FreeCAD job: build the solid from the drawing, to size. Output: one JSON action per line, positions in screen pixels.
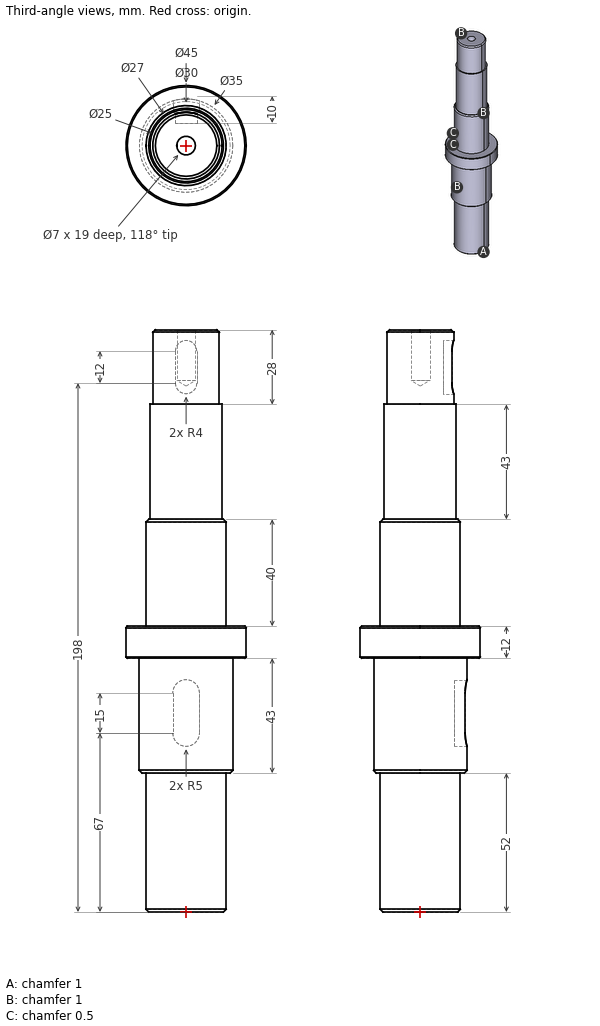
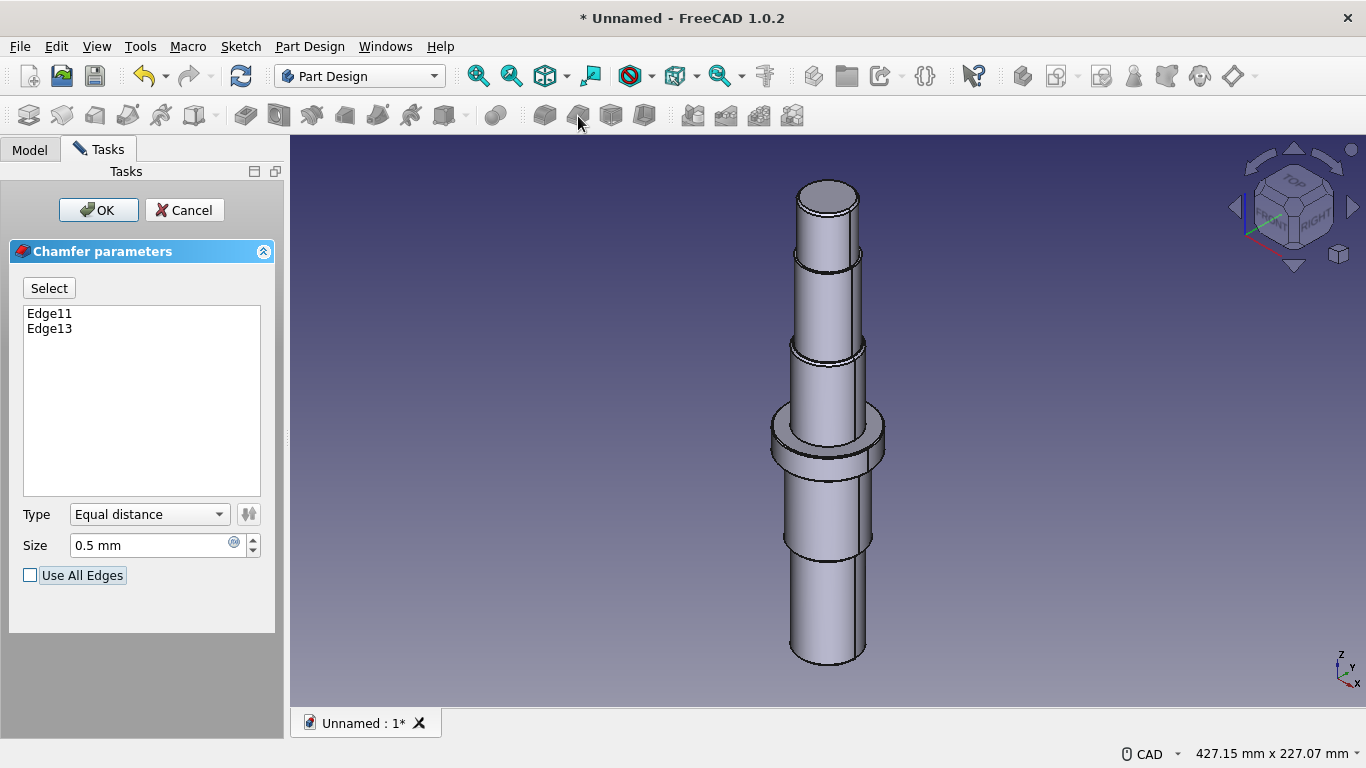
{"action": "left_click", "coordinate": [99, 210]}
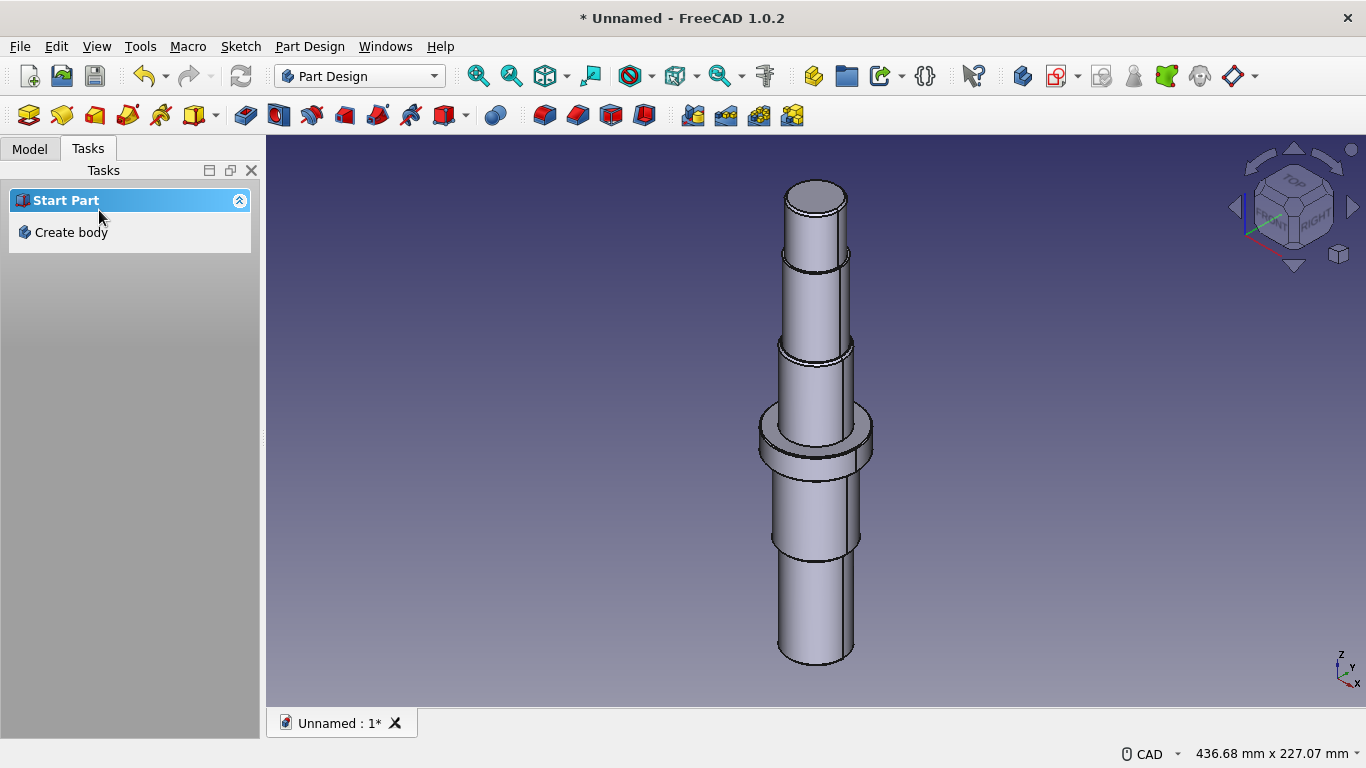
{"action": "left_click", "coordinate": [30, 148]}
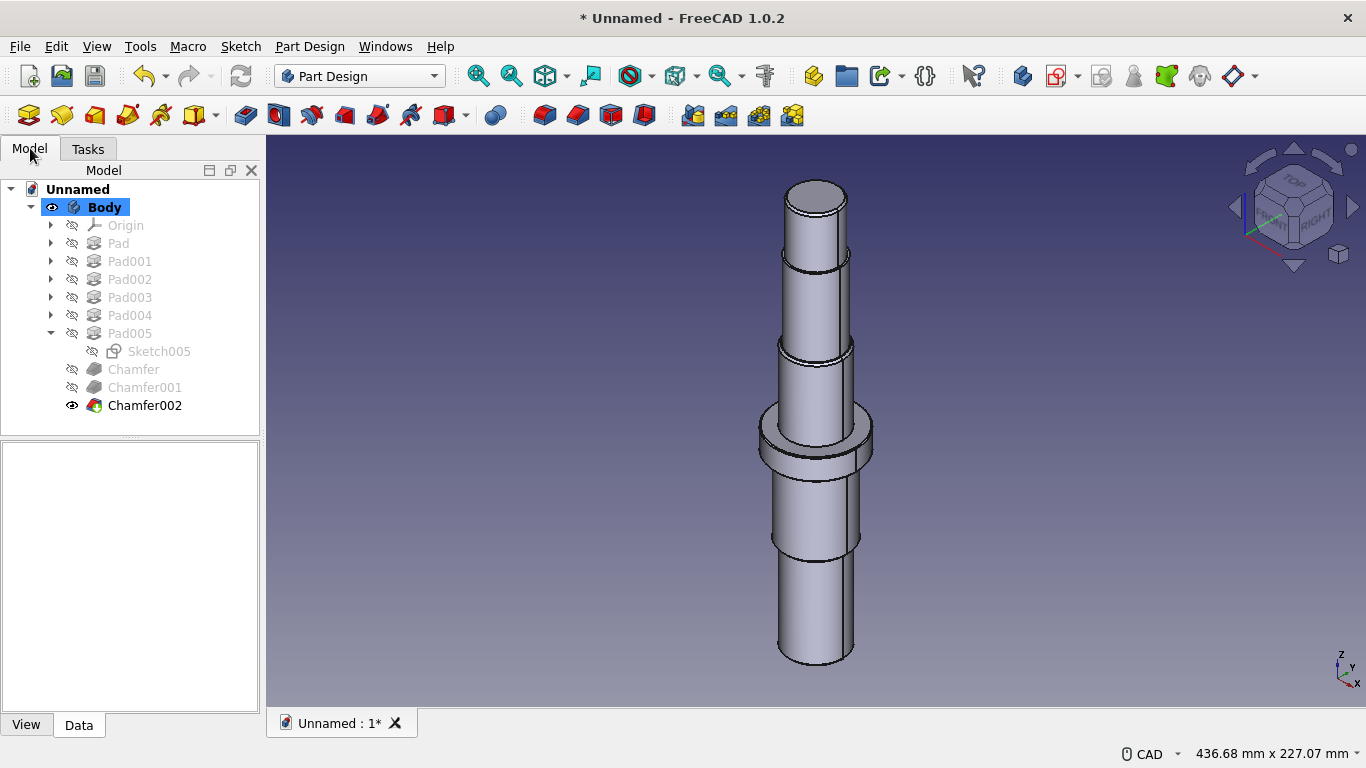
{"action": "left_click", "coordinate": [51, 225]}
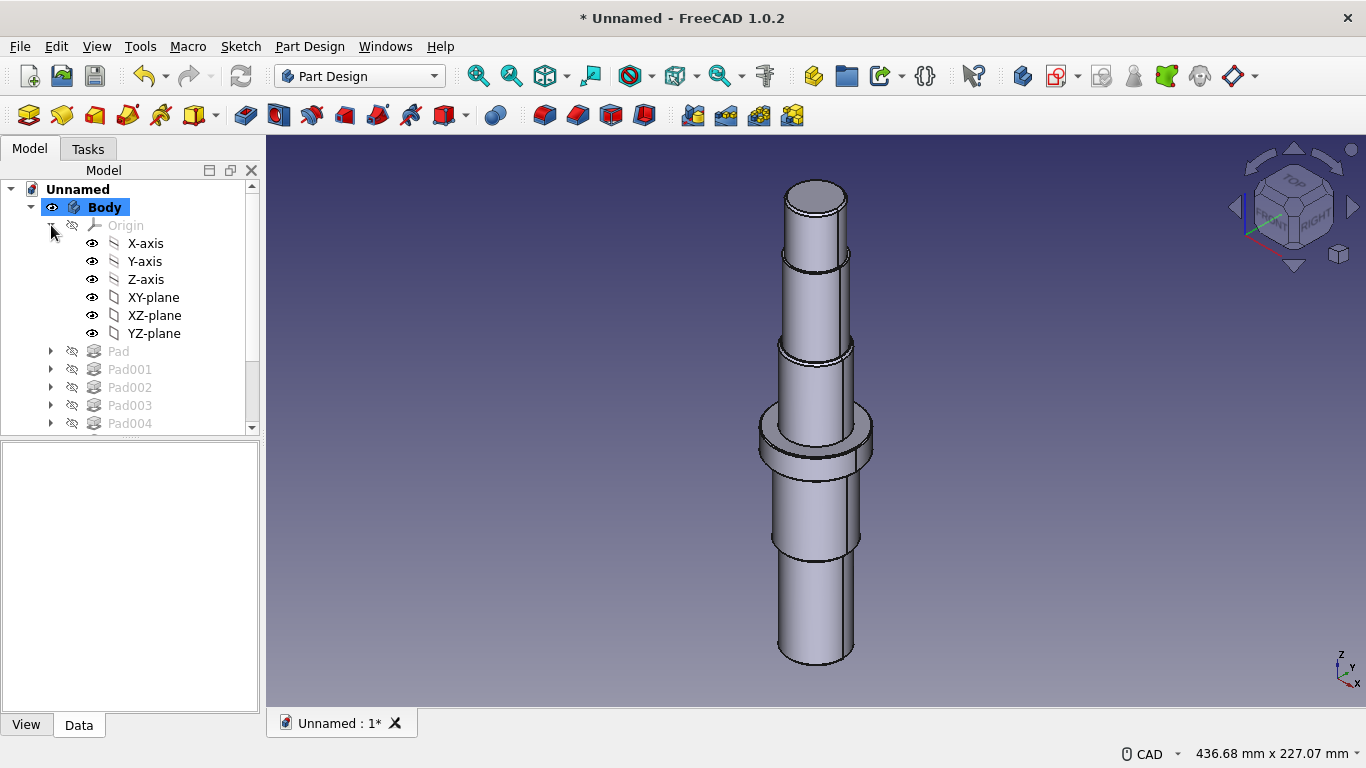
{"action": "left_click", "coordinate": [137, 315]}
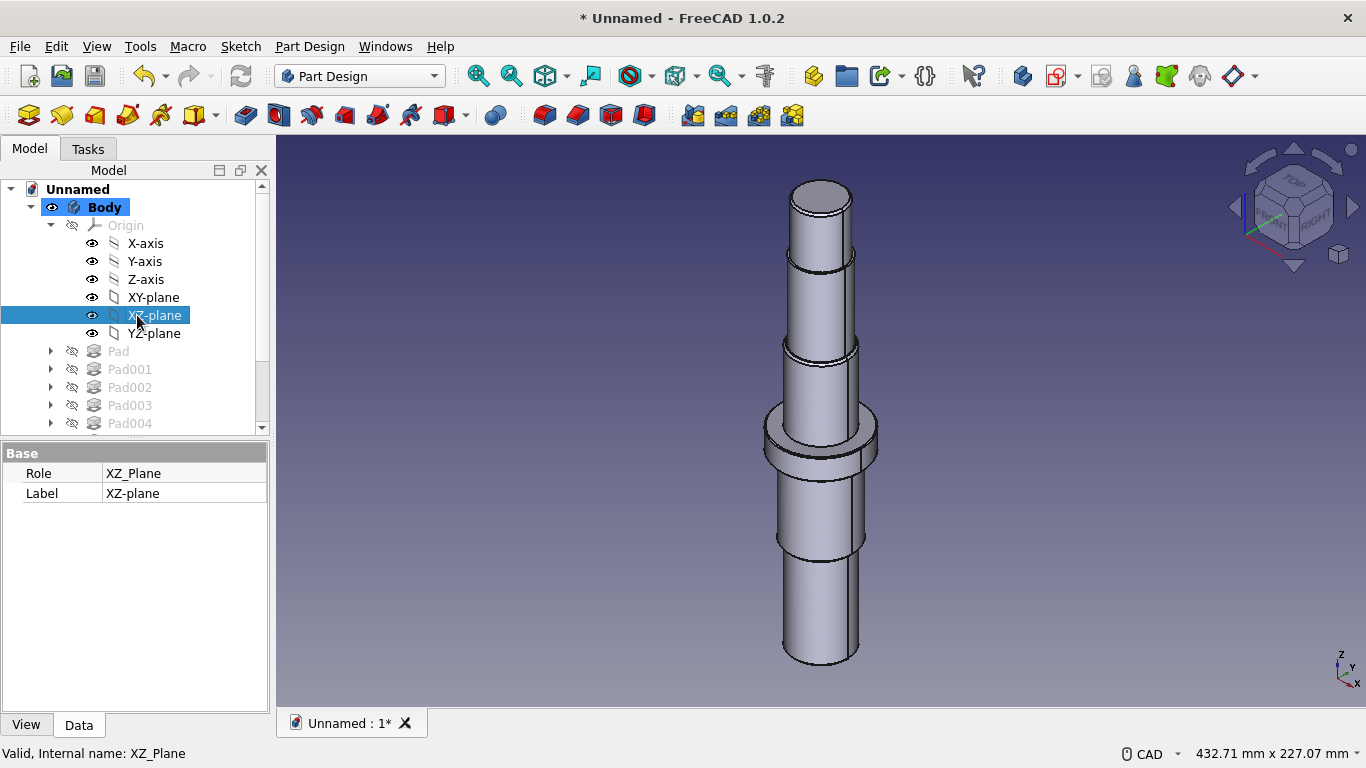
{"action": "left_click", "coordinate": [1232, 76]}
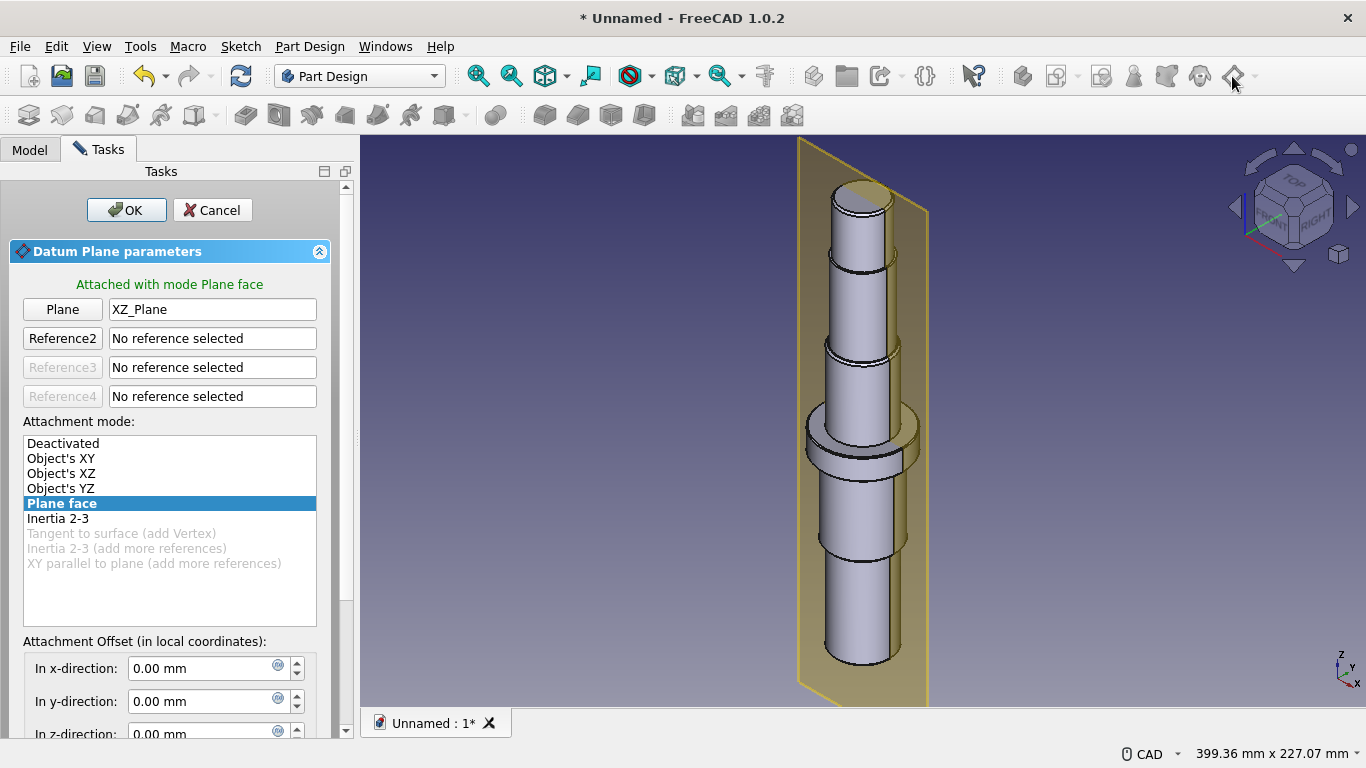
{"action": "scroll", "coordinate": [346, 460], "scroll_direction": "down", "scroll_amount": 2}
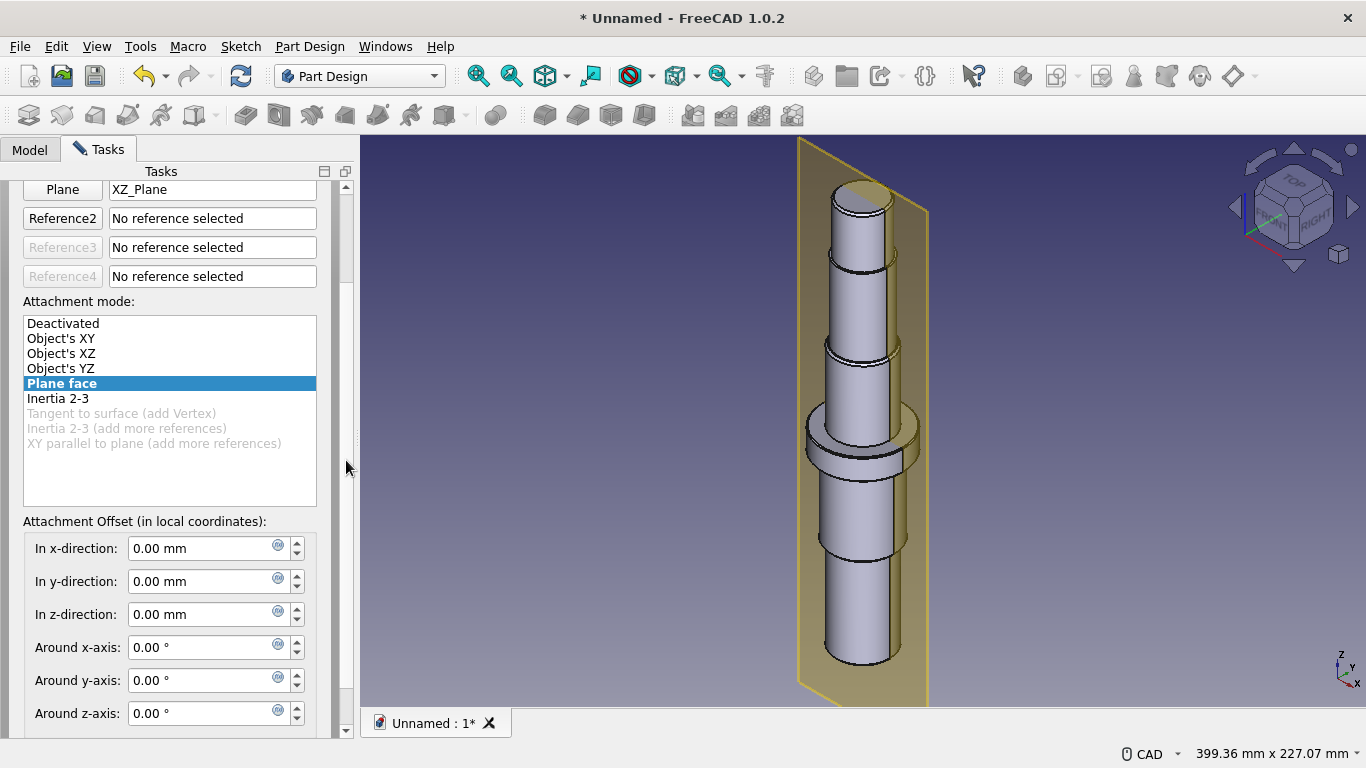
{"action": "triple_click", "coordinate": [210, 614]}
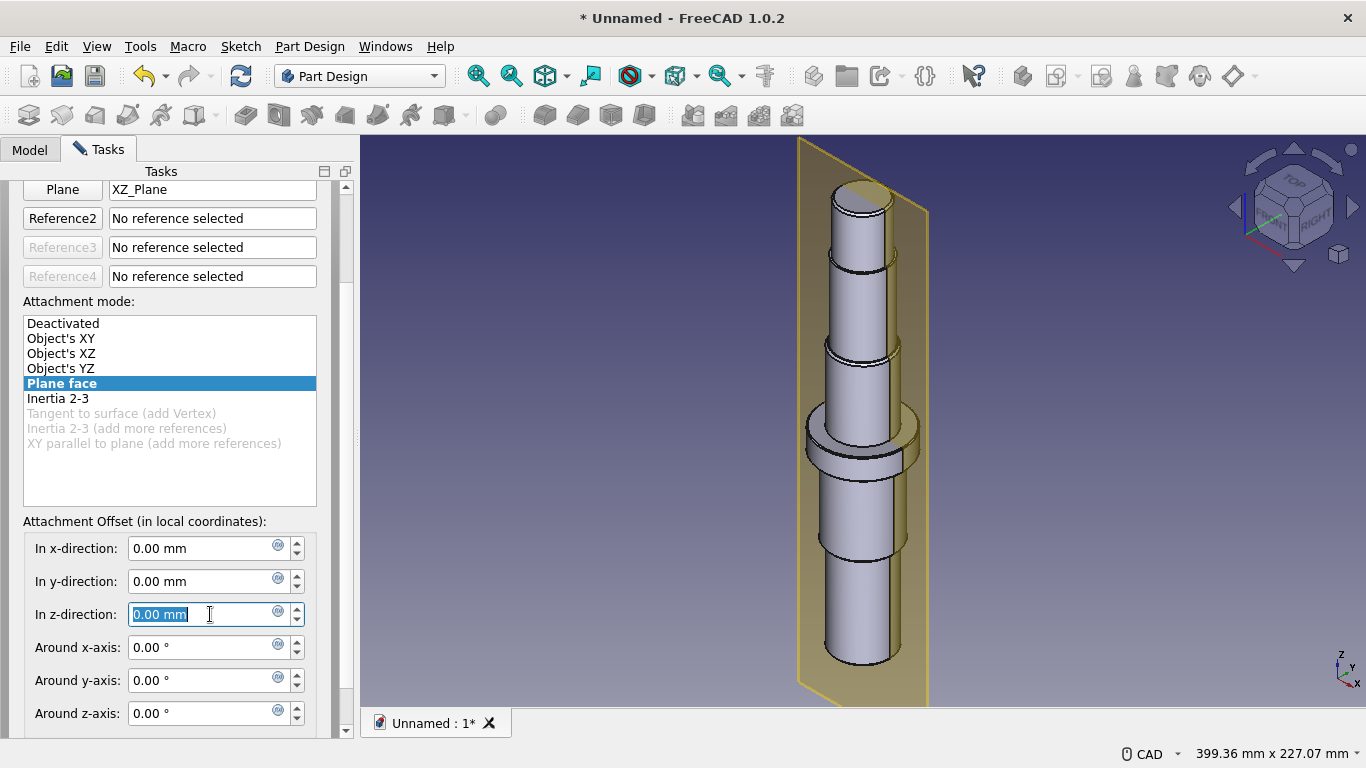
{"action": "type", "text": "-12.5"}
{"action": "key", "text": "Tab"}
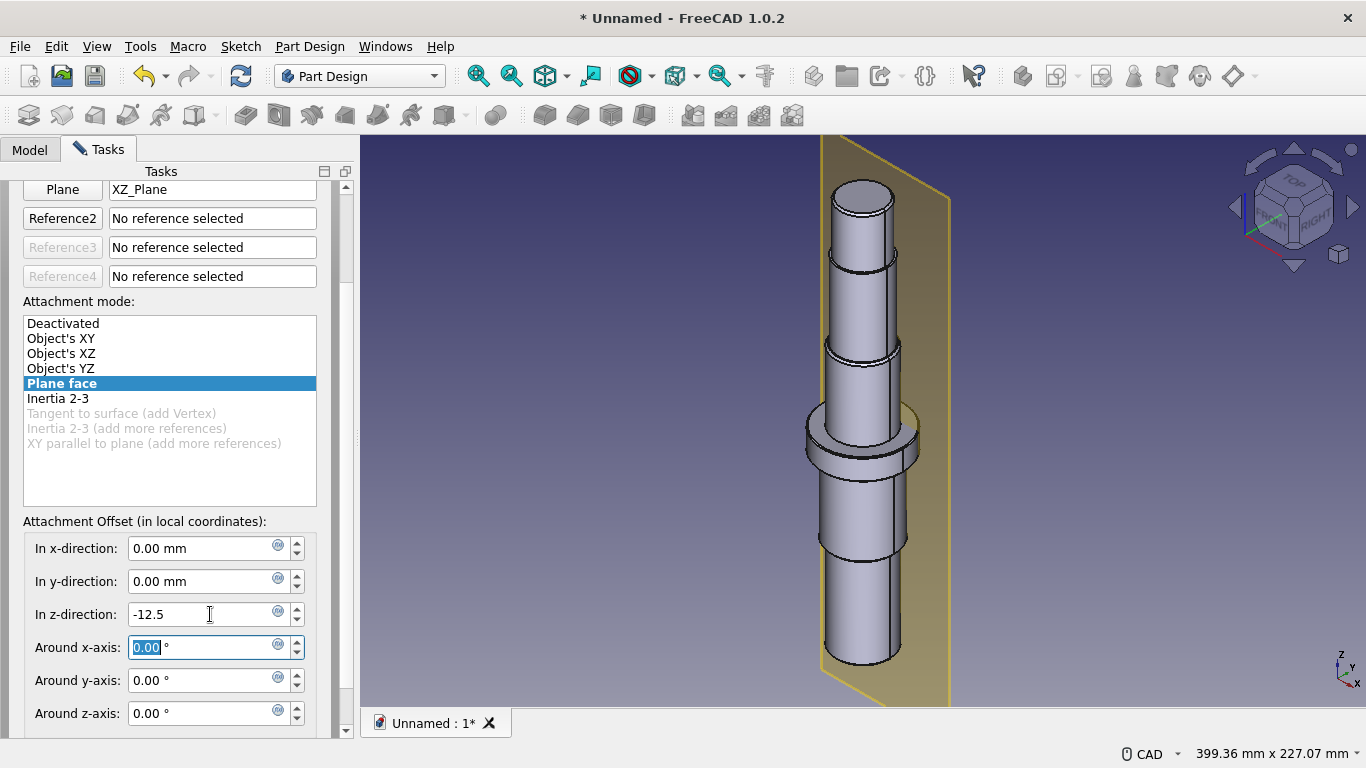
{"action": "scroll", "coordinate": [346, 460], "scroll_direction": "up", "scroll_amount": 3}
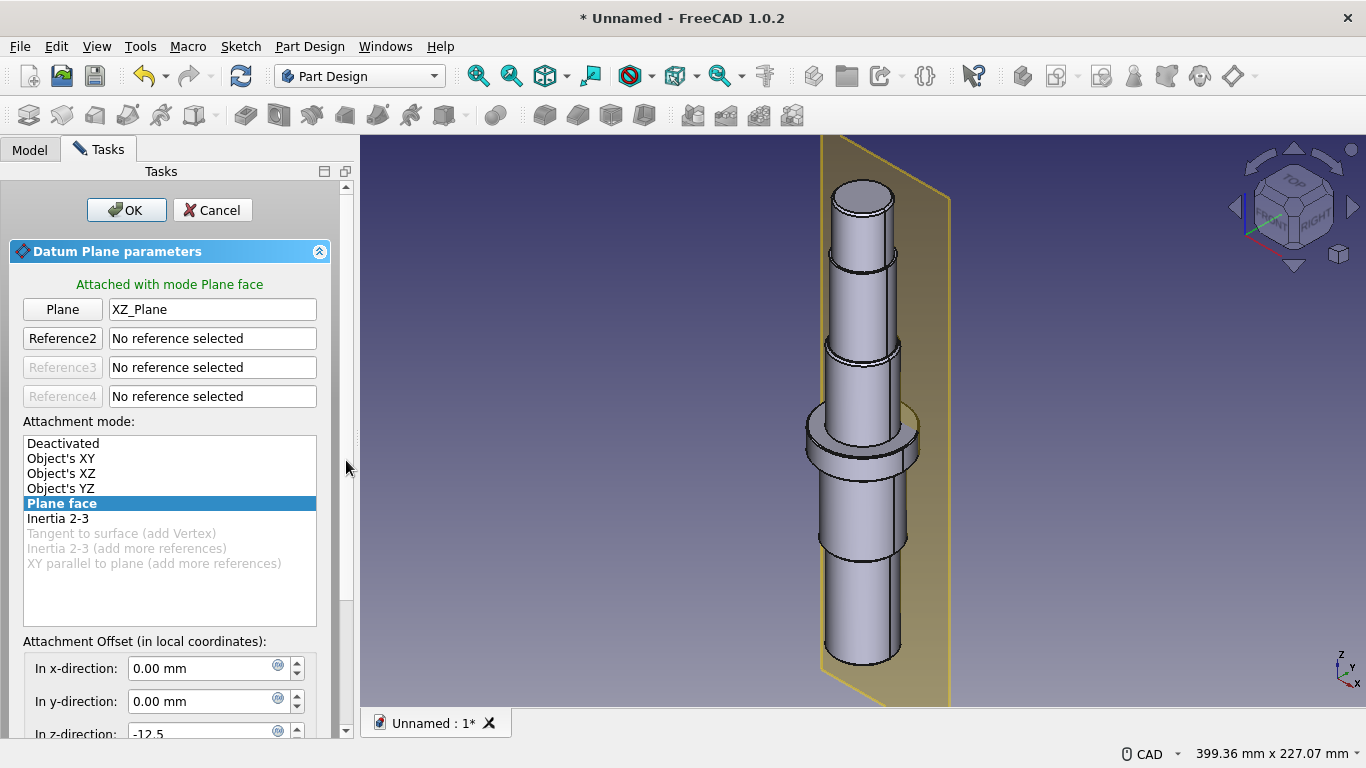
{"action": "left_click", "coordinate": [127, 210]}